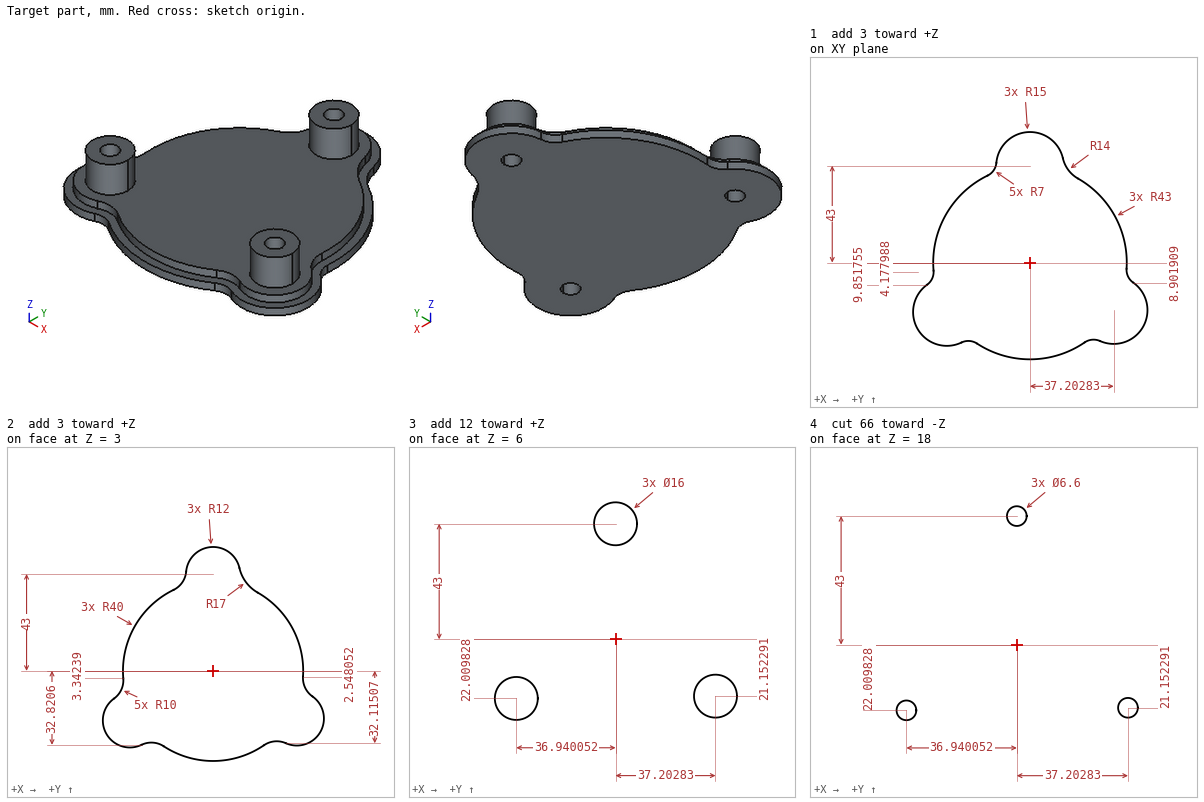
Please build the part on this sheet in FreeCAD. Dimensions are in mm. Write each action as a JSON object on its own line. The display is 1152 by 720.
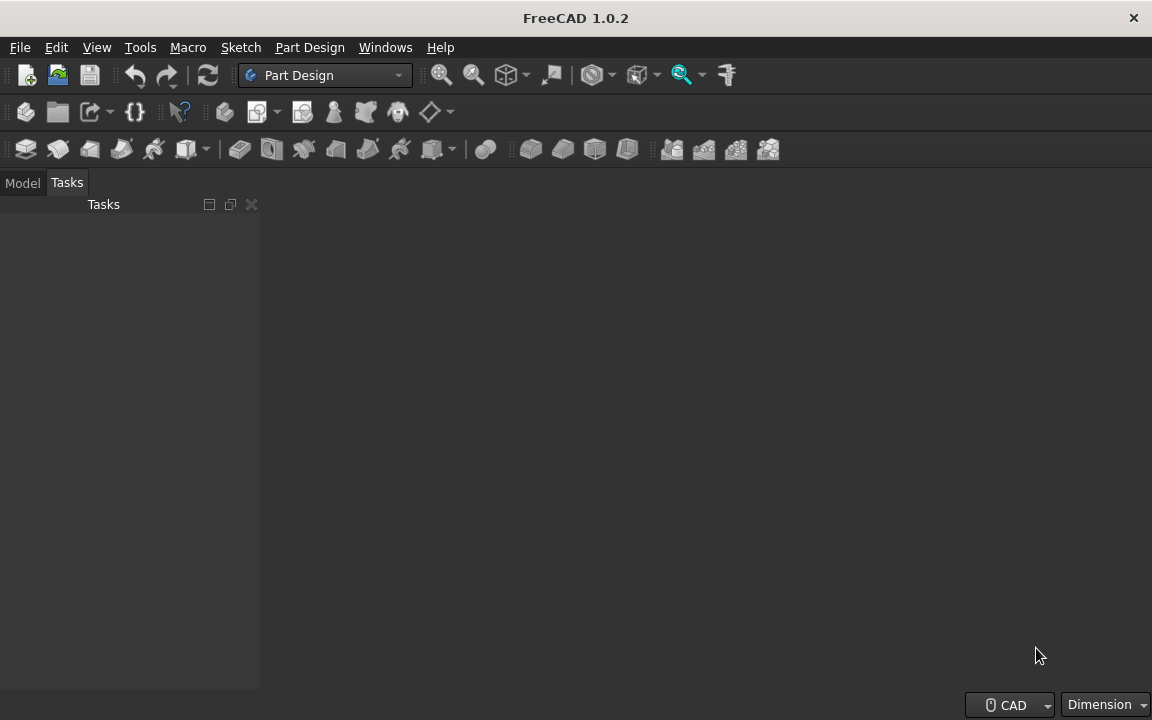
{"action": "left_click", "coordinate": [26, 76]}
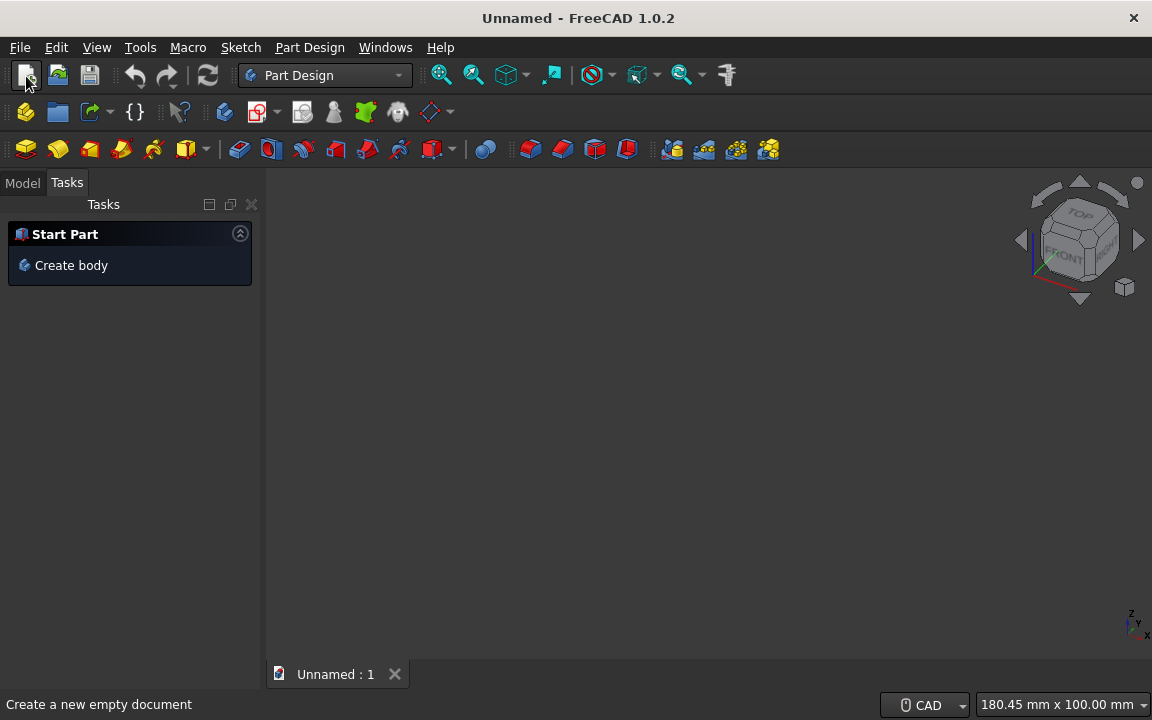
{"action": "left_click", "coordinate": [258, 112]}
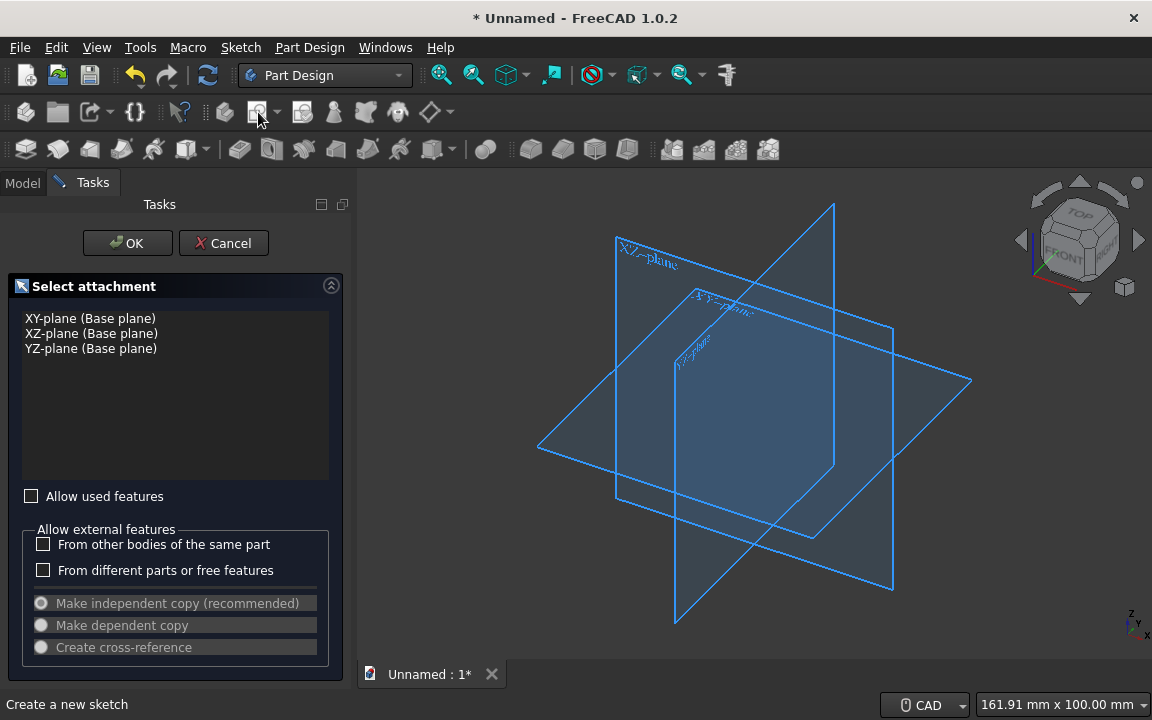
{"action": "left_click", "coordinate": [82, 318]}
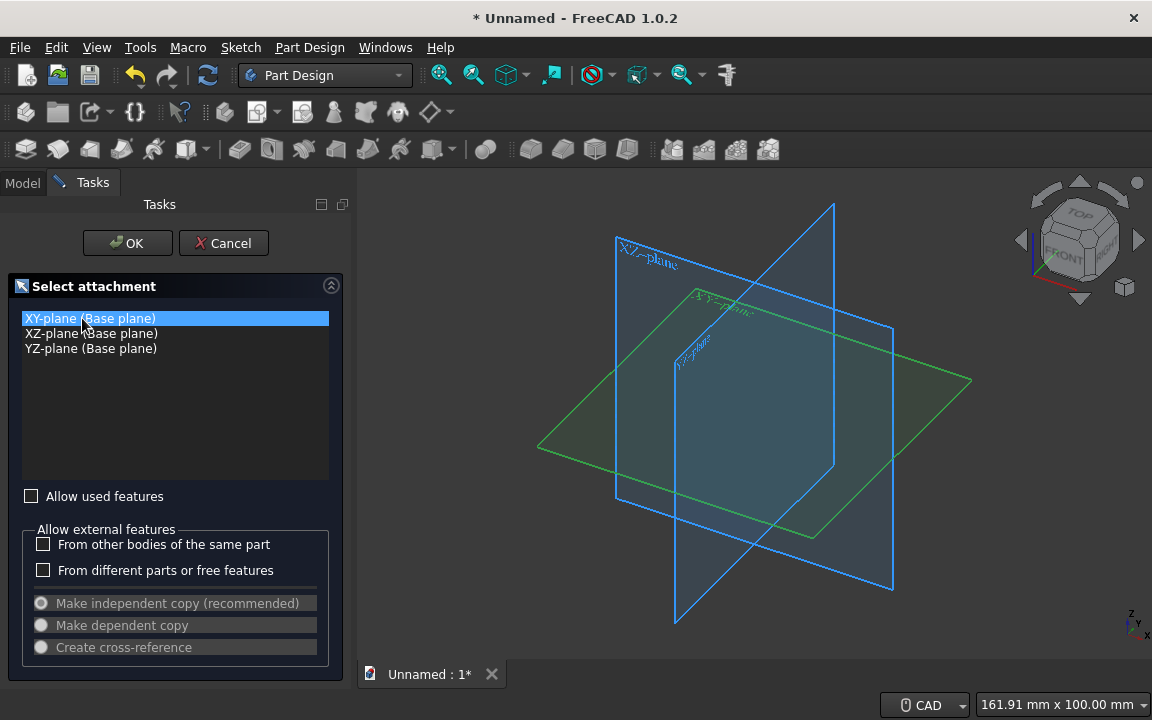
{"action": "left_click", "coordinate": [128, 243]}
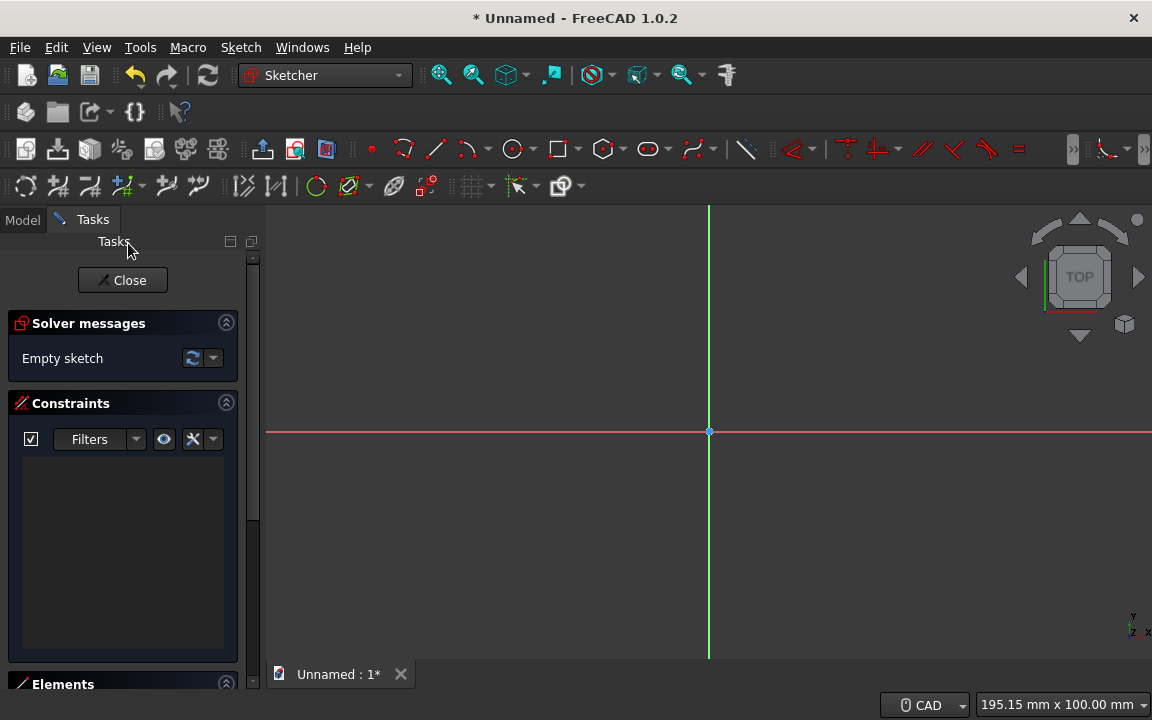
{"action": "scroll", "coordinate": [499, 501], "scroll_direction": "down", "scroll_amount": 2}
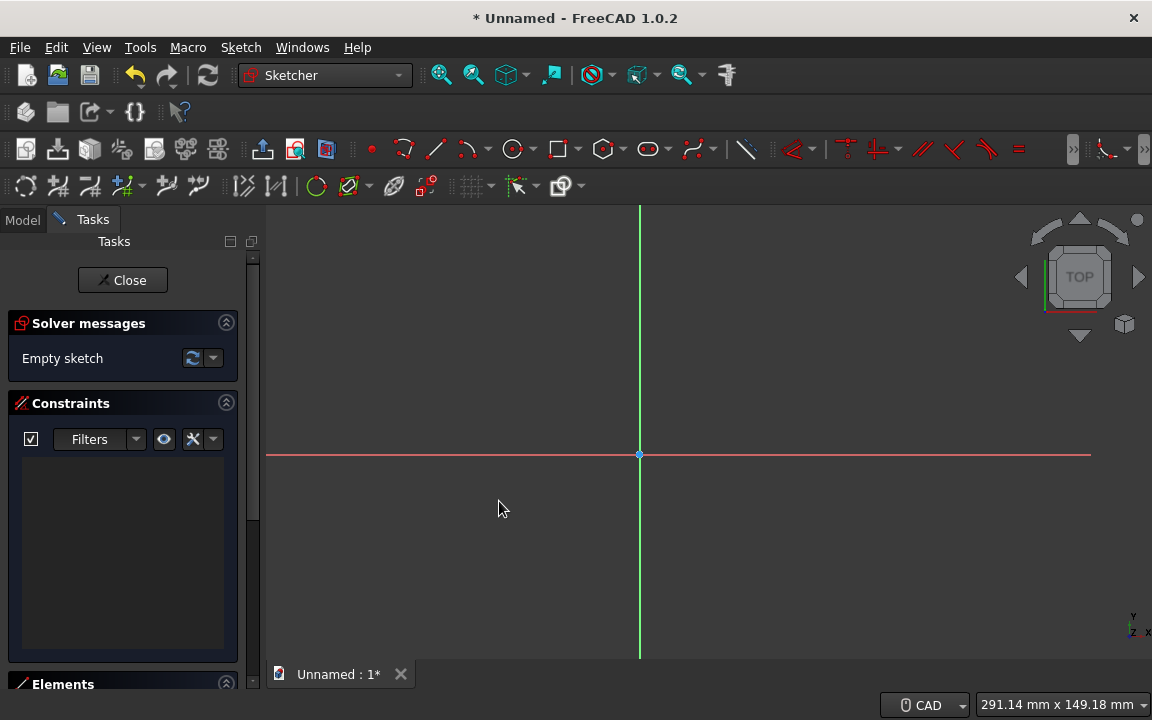
{"action": "key", "text": "g 3 a"}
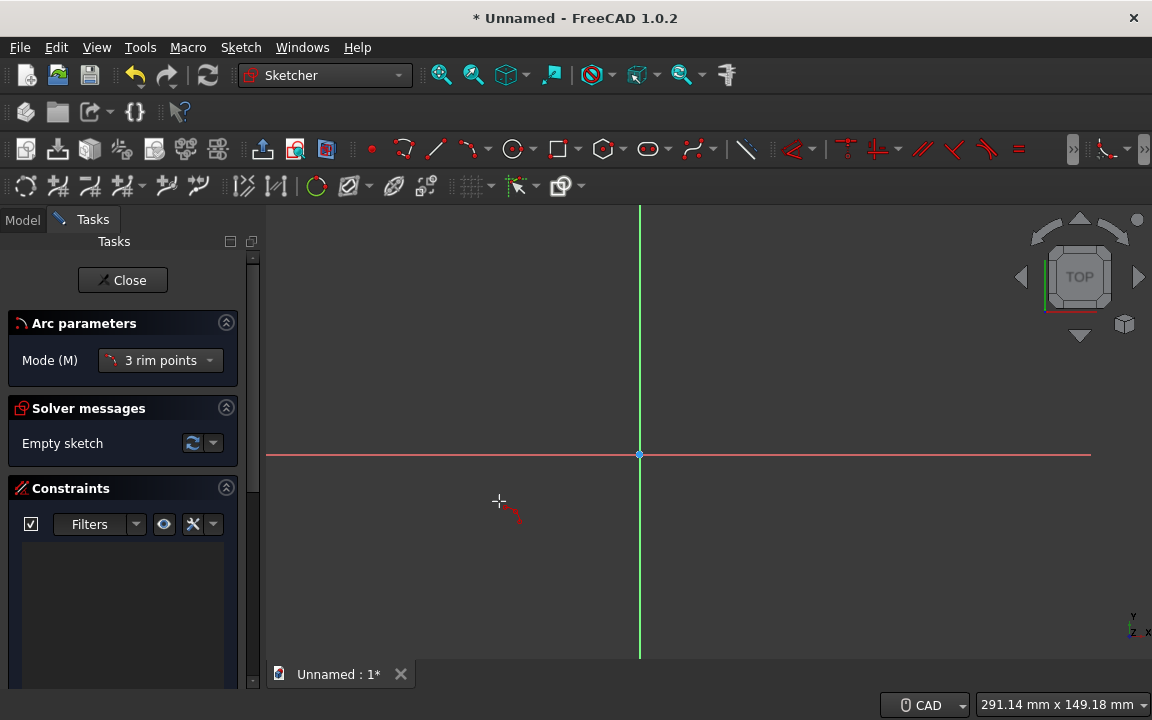
{"action": "scroll", "coordinate": [509, 466], "scroll_direction": "up", "scroll_amount": 2}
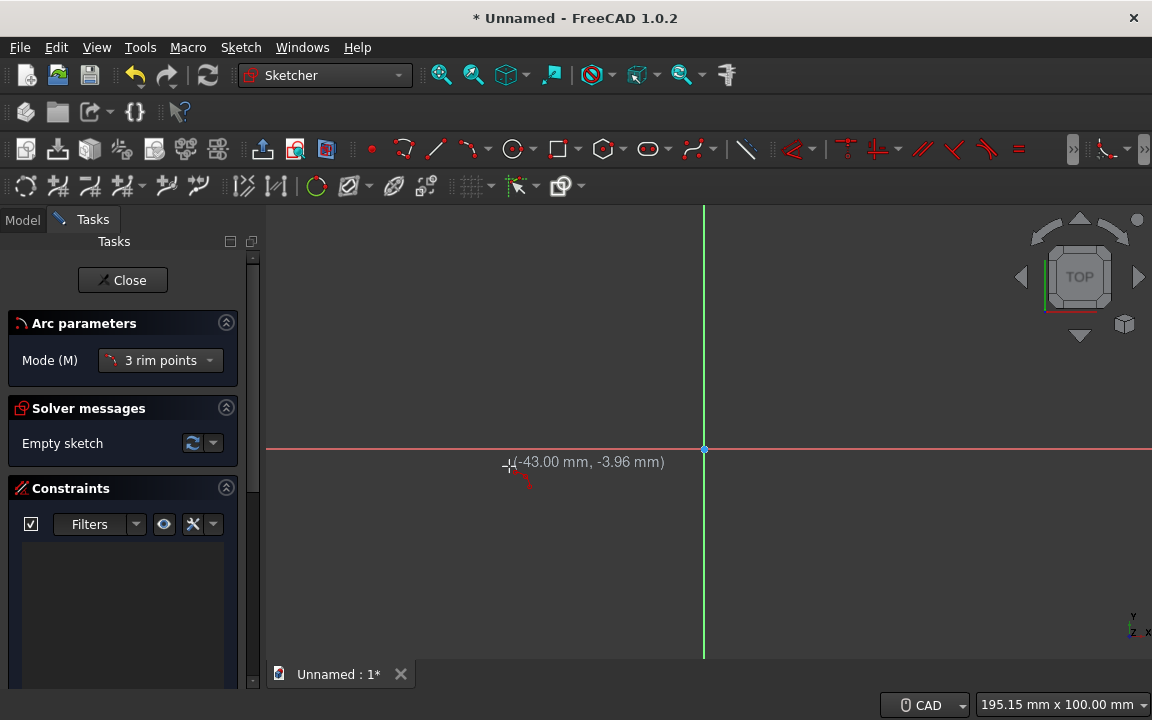
{"action": "left_click", "coordinate": [510, 466]}
{"action": "left_click", "coordinate": [496, 494]}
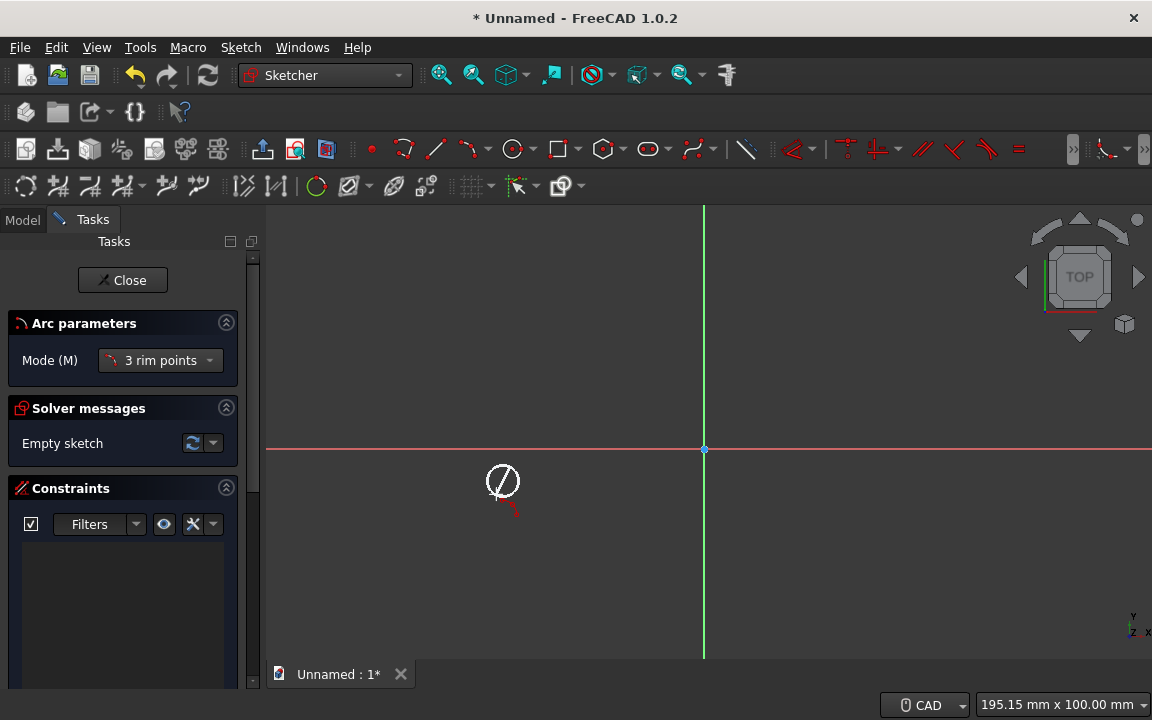
{"action": "scroll", "coordinate": [507, 481], "scroll_direction": "up", "scroll_amount": 7}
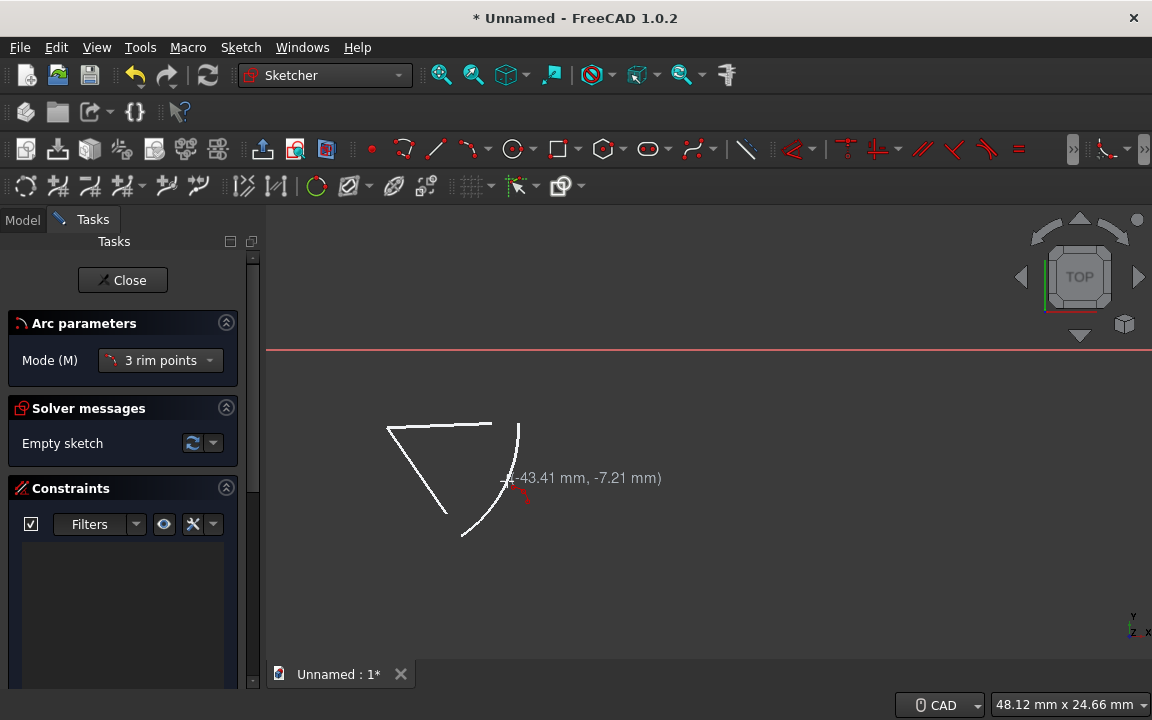
{"action": "left_click", "coordinate": [505, 481]}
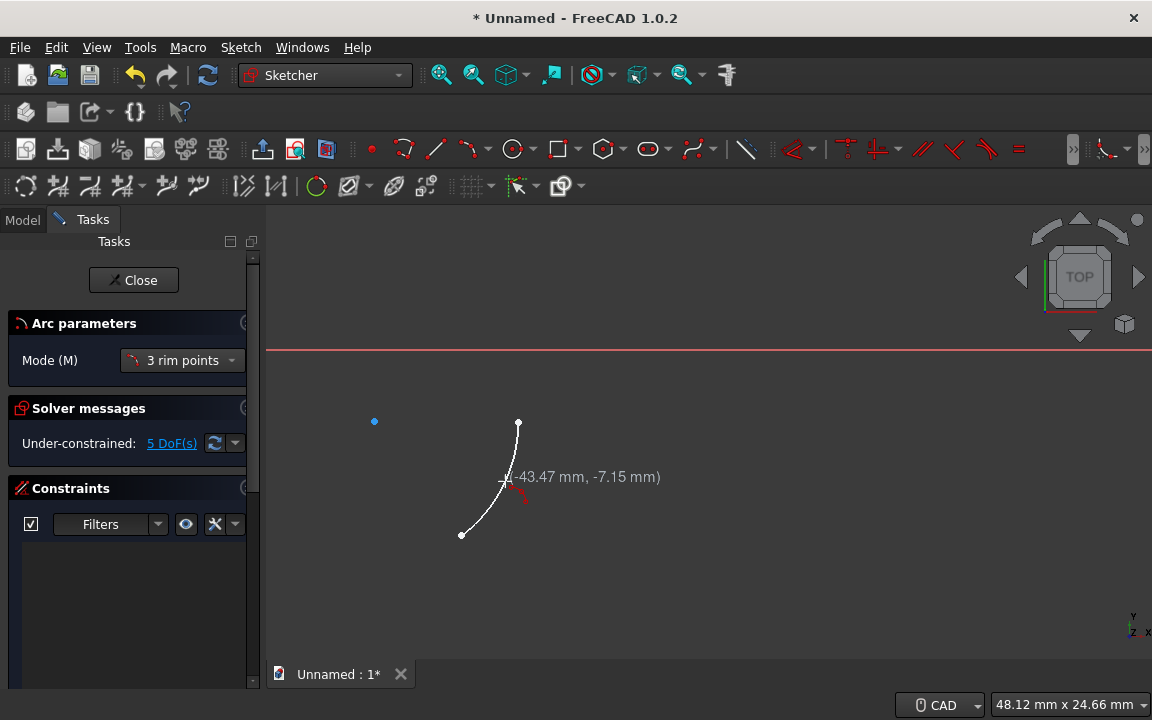
{"action": "scroll", "coordinate": [508, 475], "scroll_direction": "down", "scroll_amount": 9}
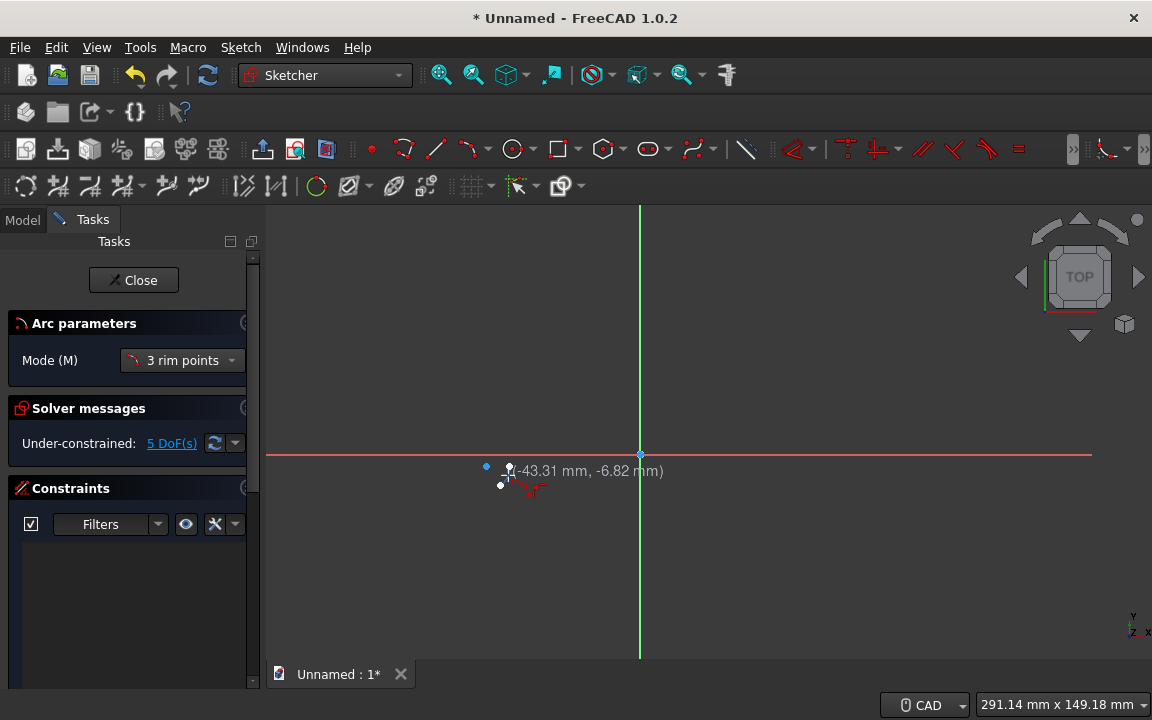
{"action": "left_click", "coordinate": [501, 486]}
{"action": "left_click", "coordinate": [547, 563]}
{"action": "left_click", "coordinate": [488, 545]}